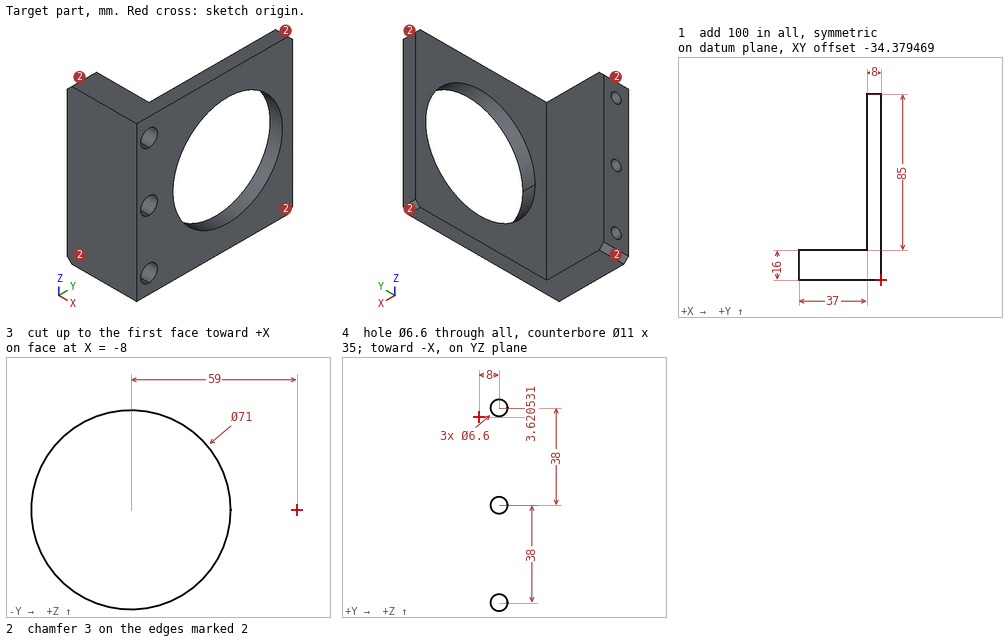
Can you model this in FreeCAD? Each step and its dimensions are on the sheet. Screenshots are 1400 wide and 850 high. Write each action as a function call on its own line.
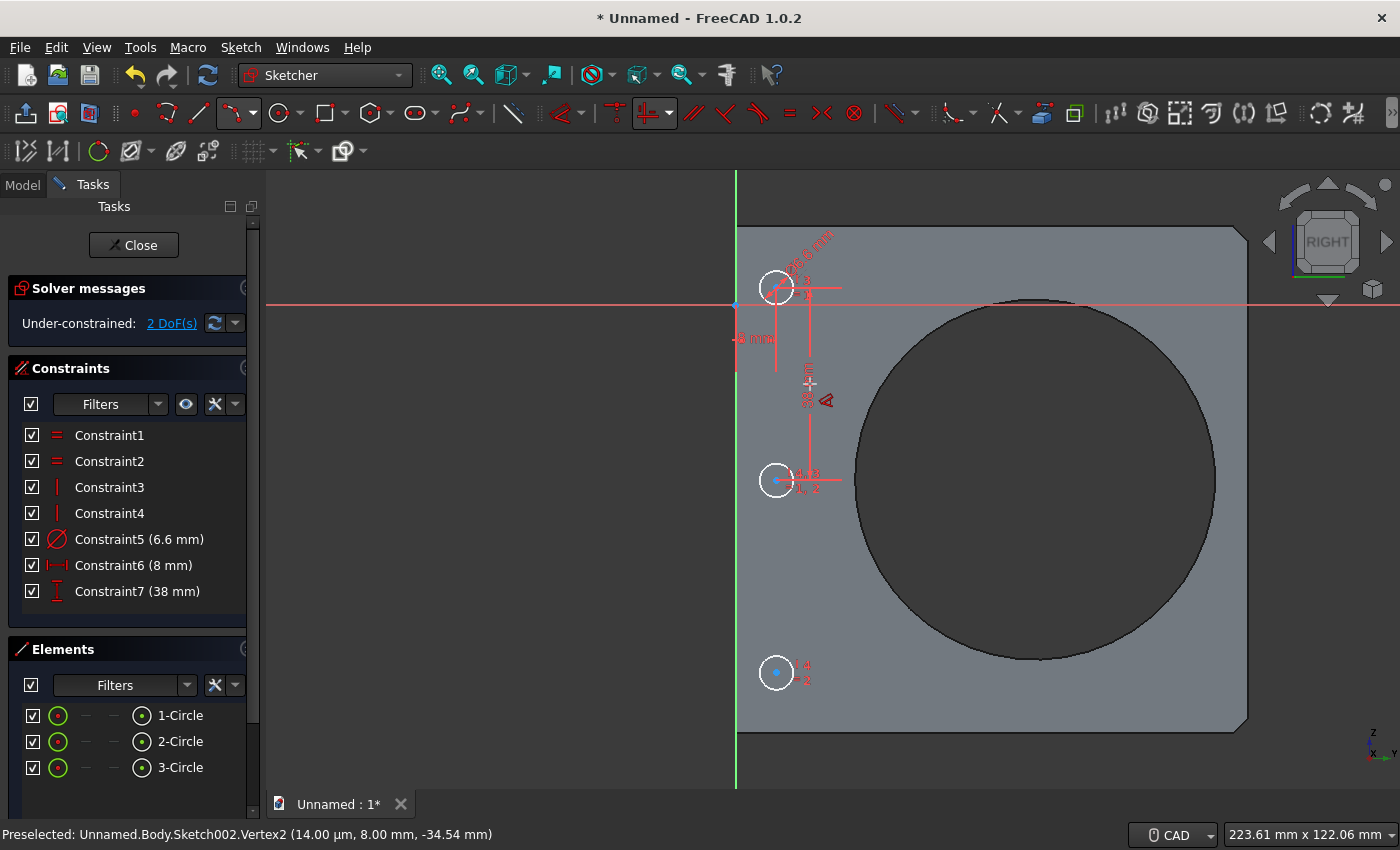
click(776, 480)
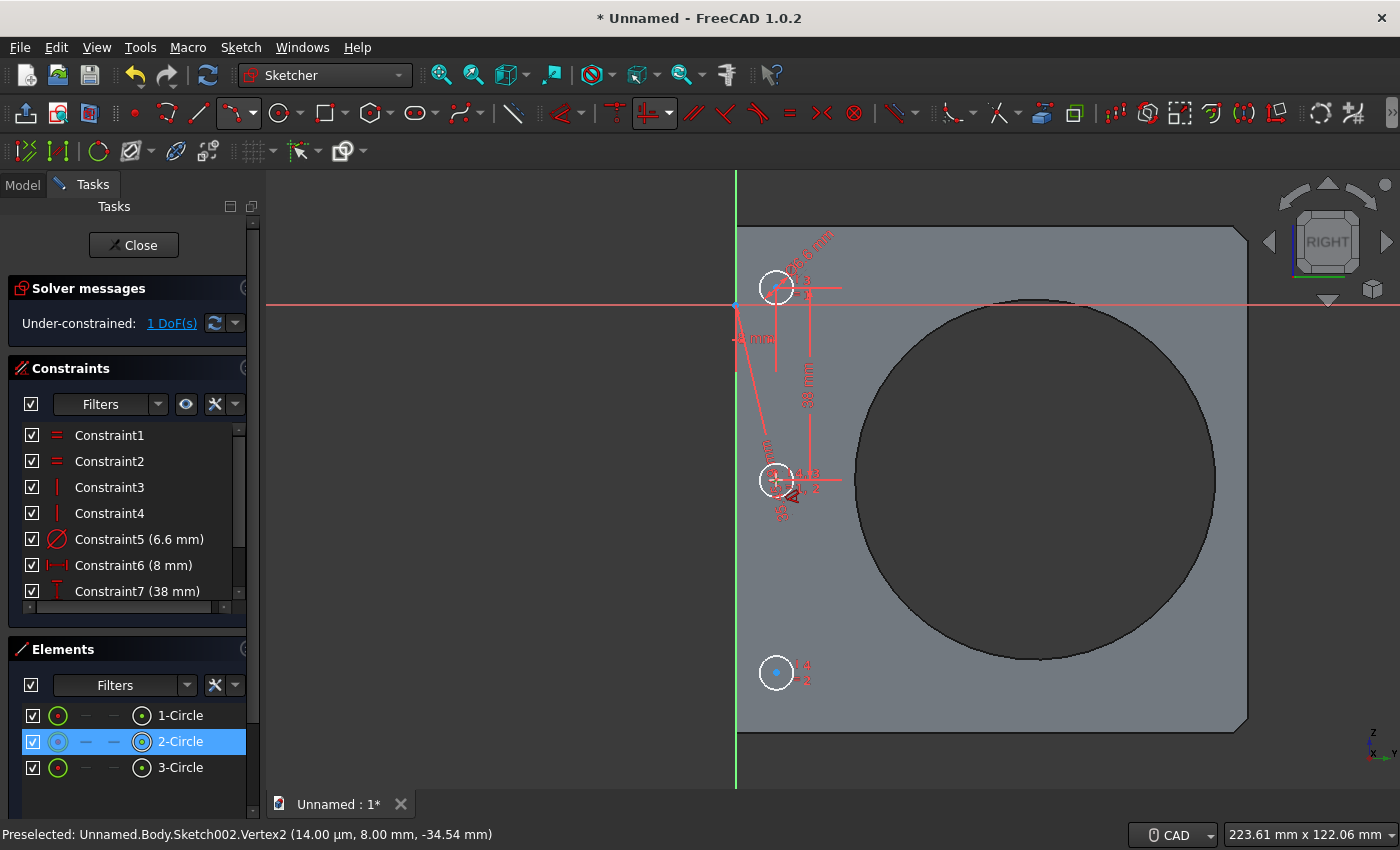
click(776, 673)
click(810, 577)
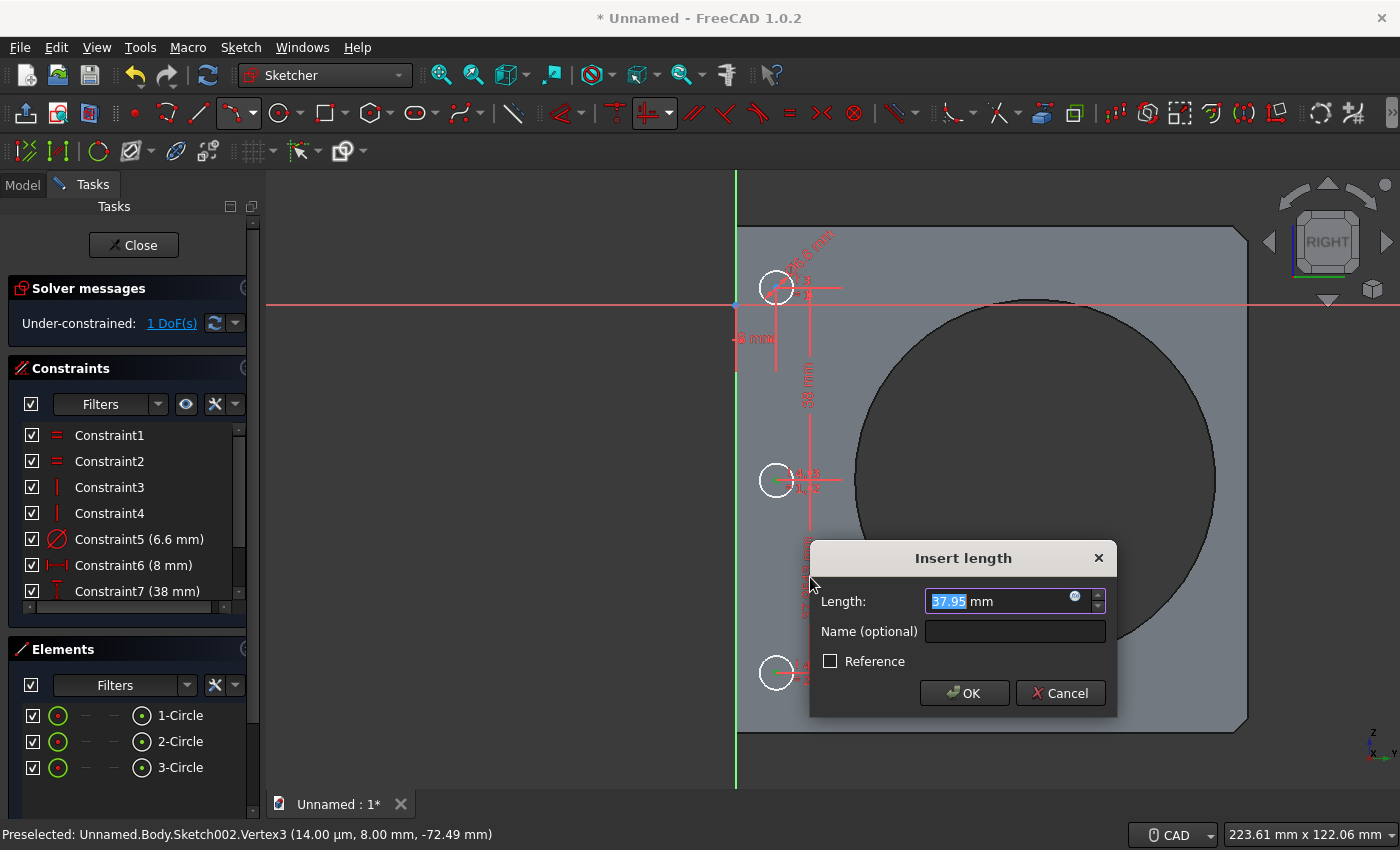
text(38)
key(Return)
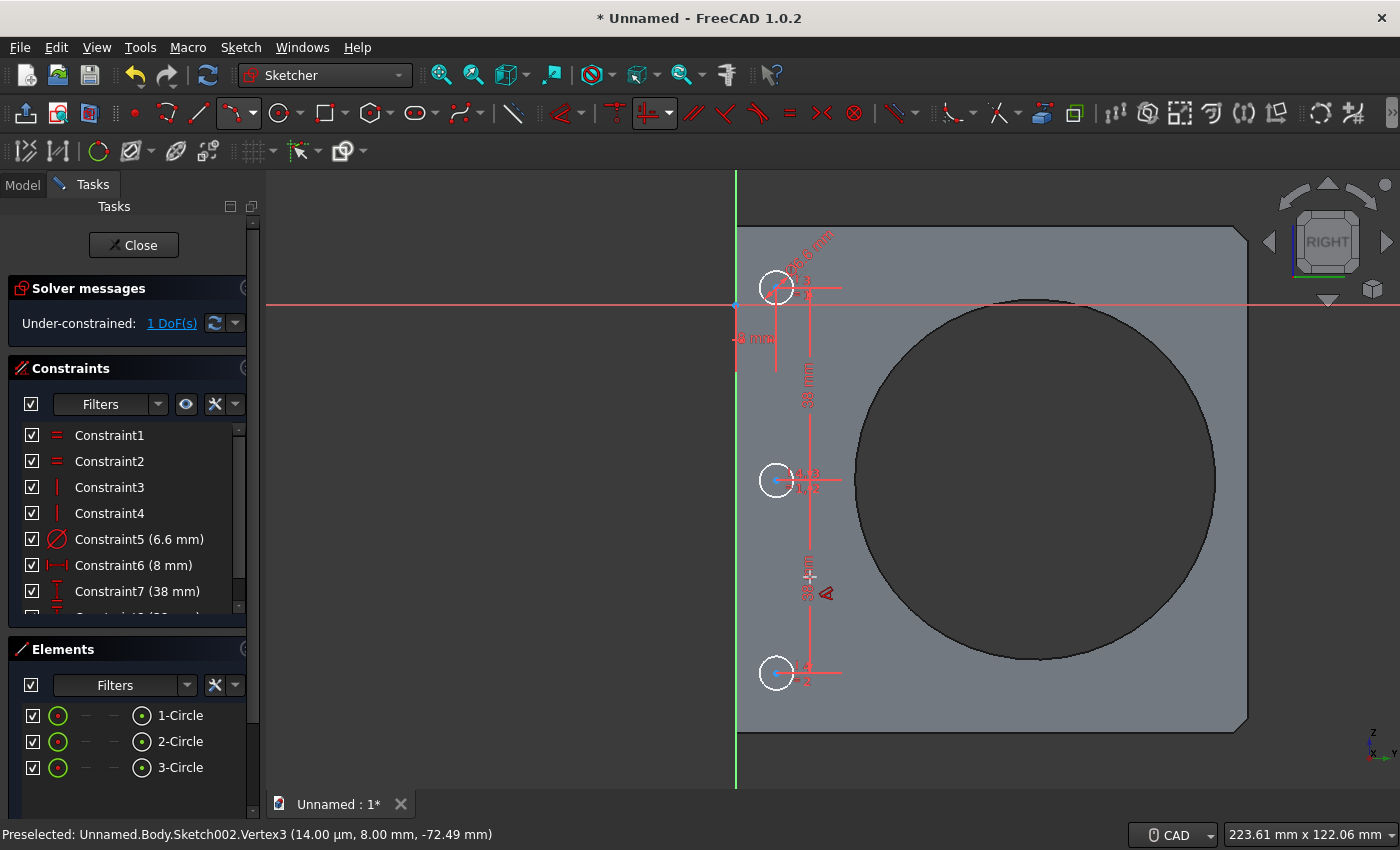
scroll(776, 288, up, 4)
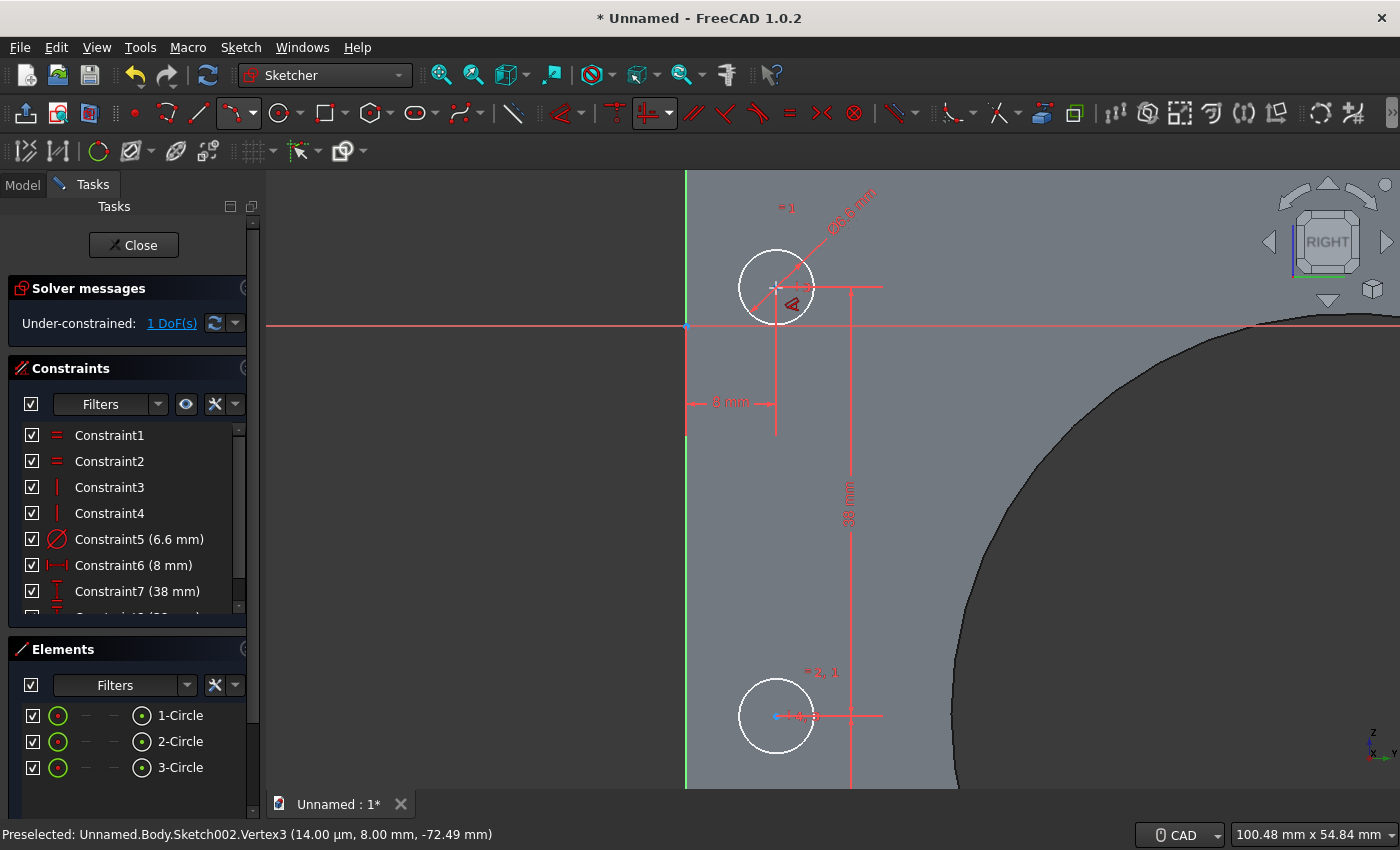
click(776, 287)
click(652, 307)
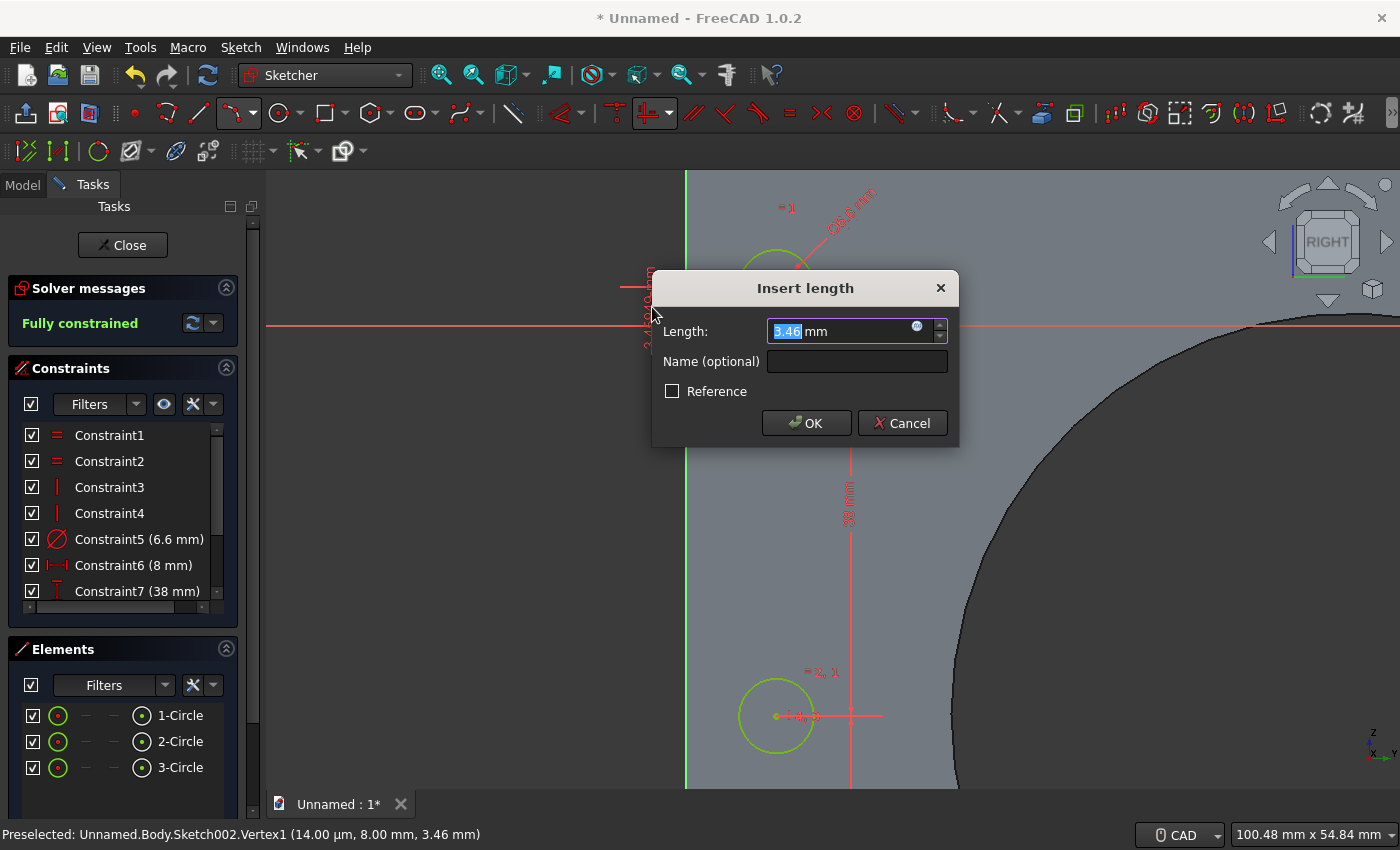
text(3.620531)
key(Return)
key(Escape)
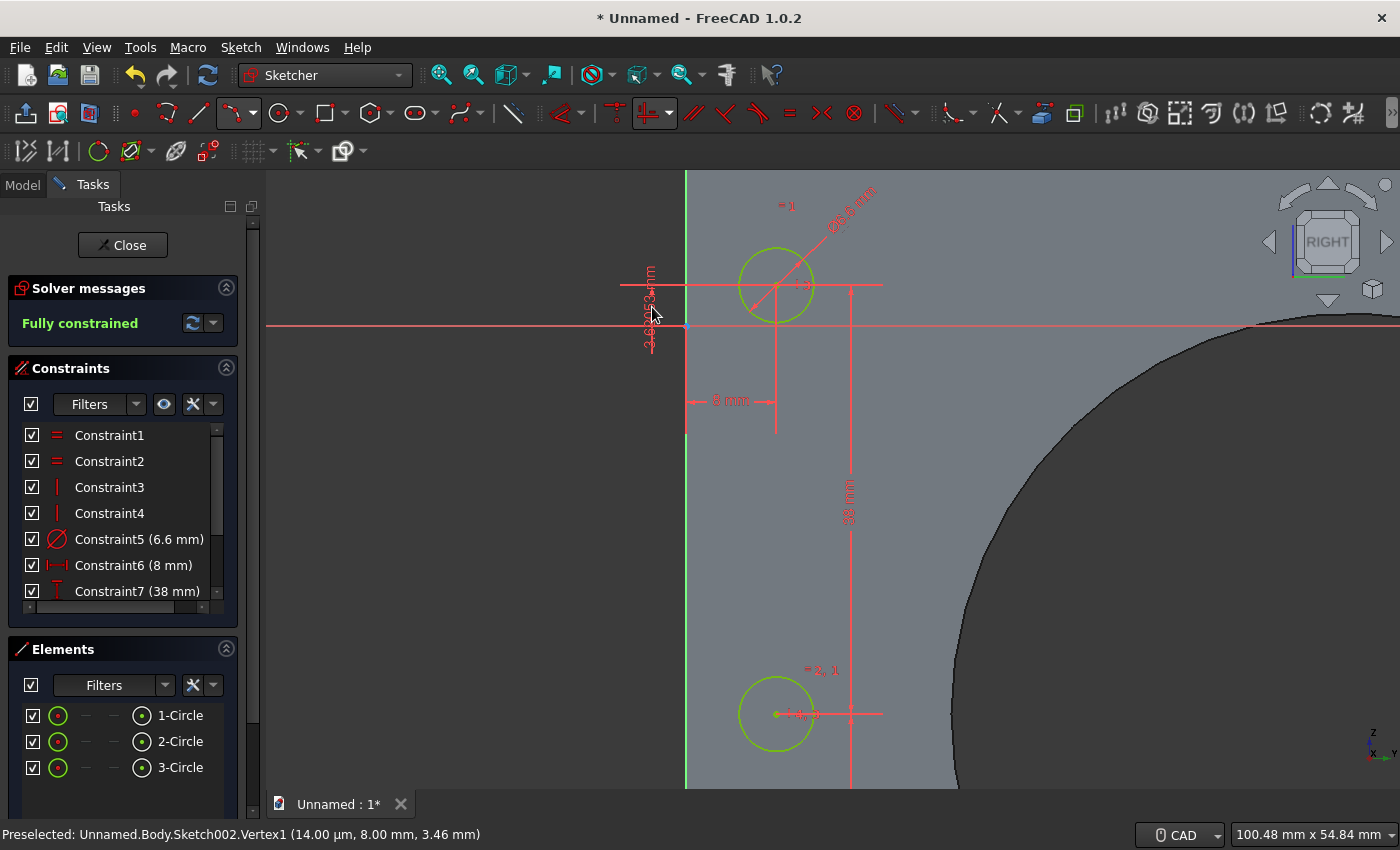
click(123, 245)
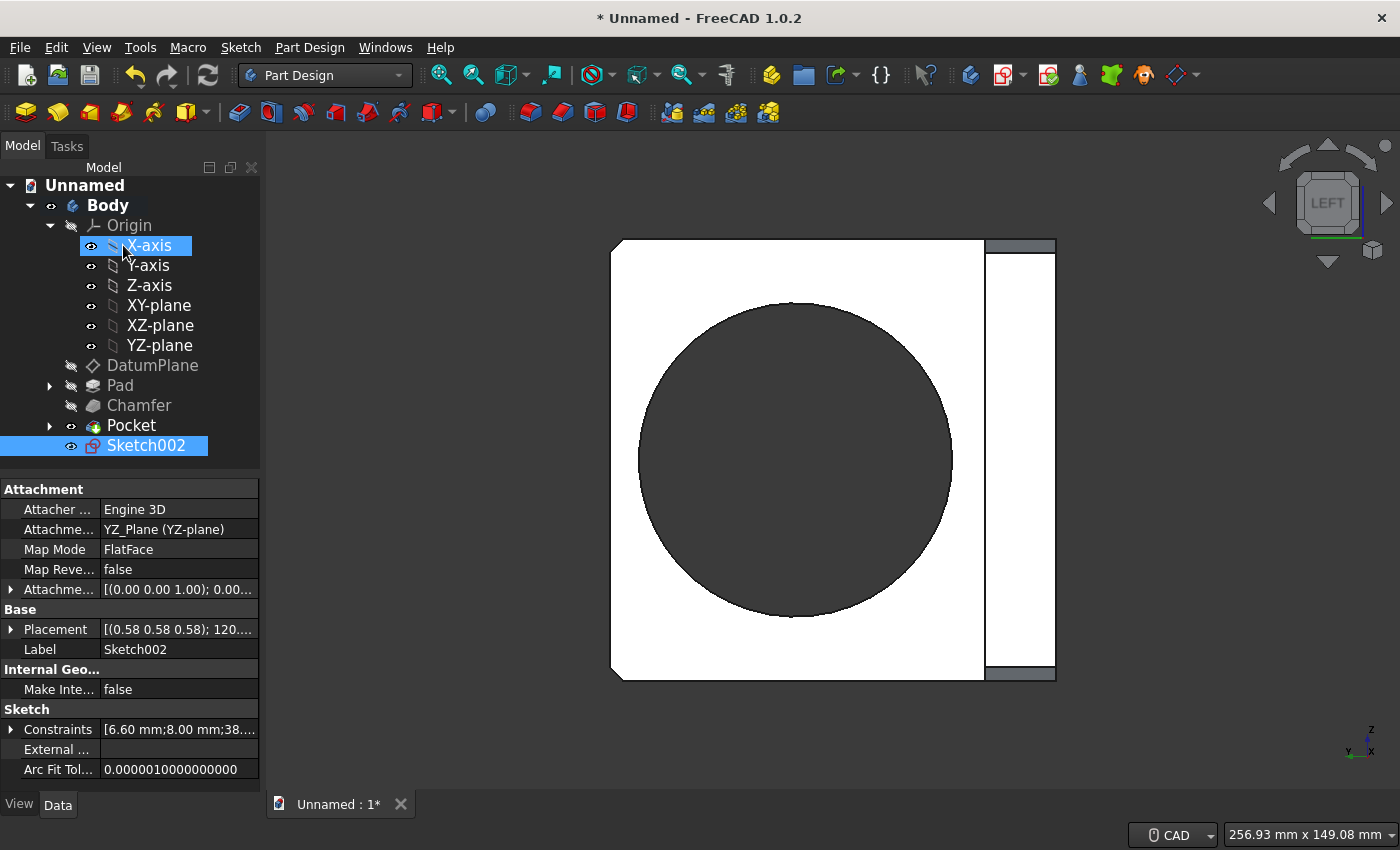
click(272, 112)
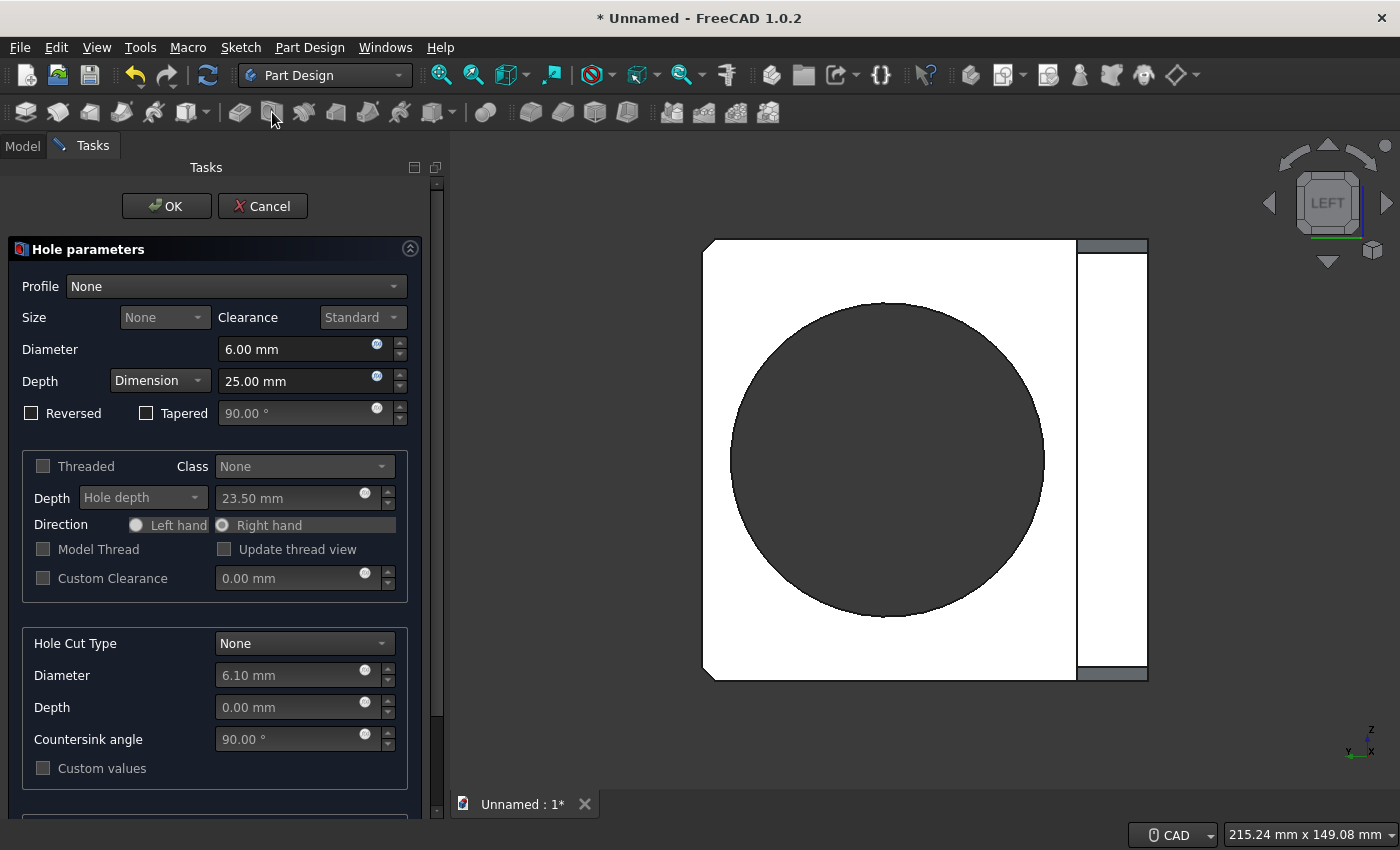
triple_click(305, 349)